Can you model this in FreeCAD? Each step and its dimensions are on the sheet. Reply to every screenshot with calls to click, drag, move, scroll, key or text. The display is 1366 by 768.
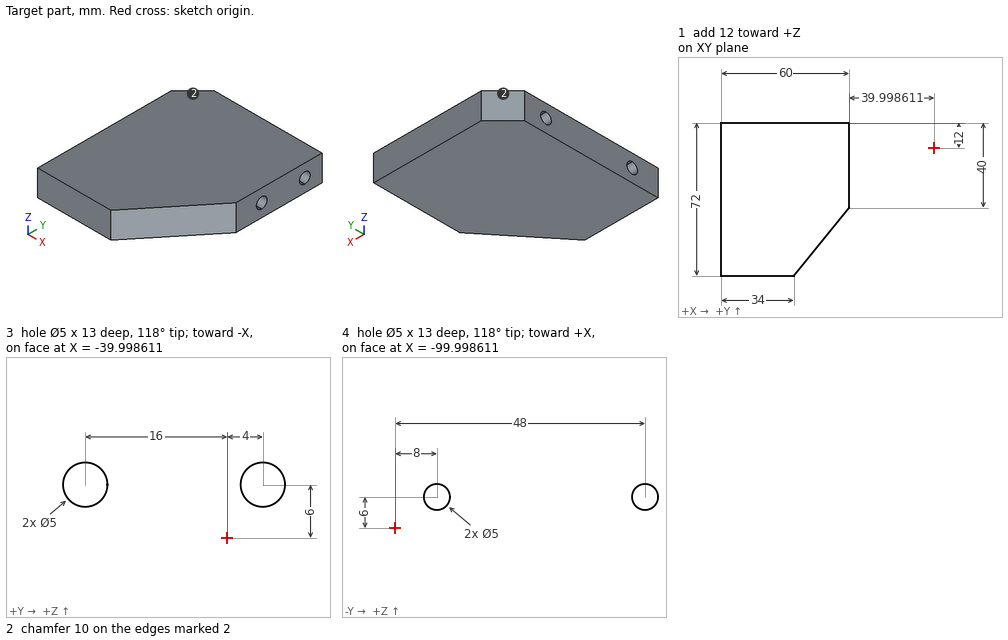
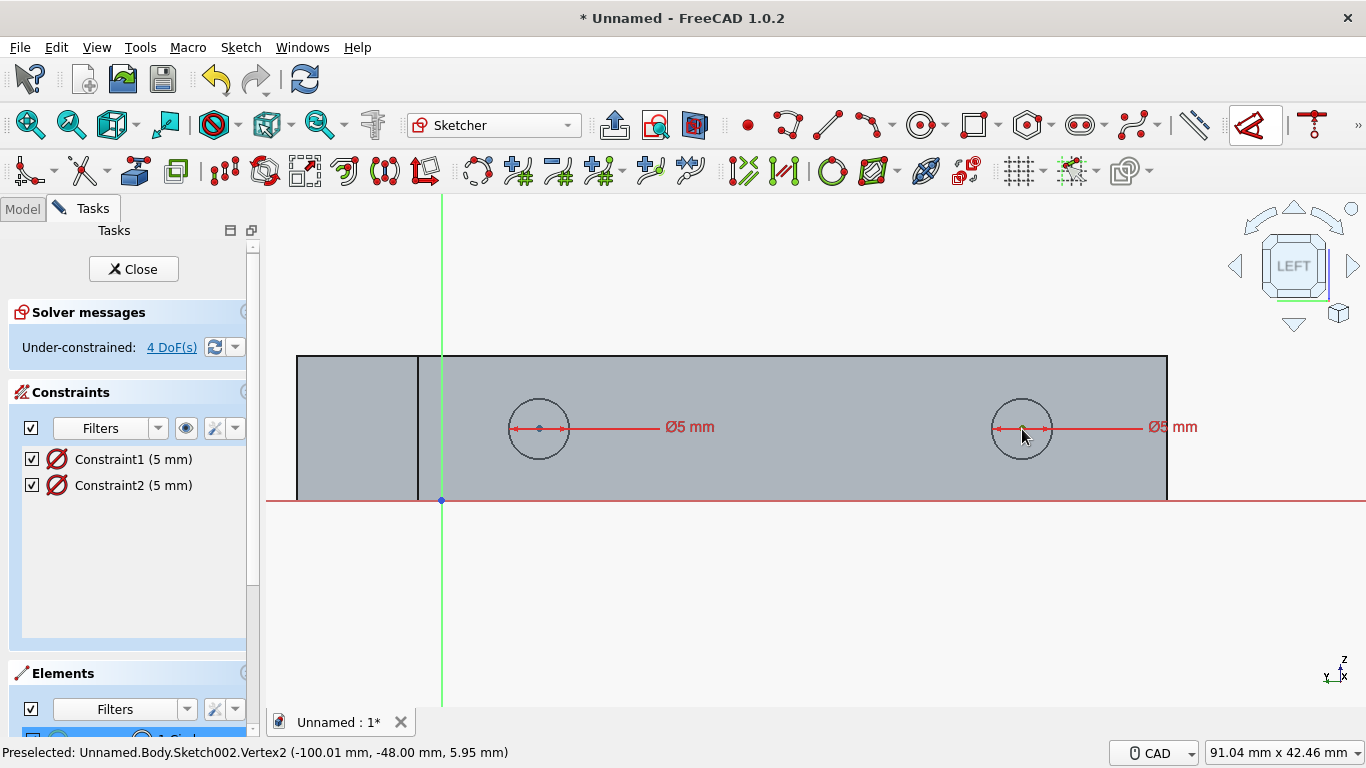
key(h)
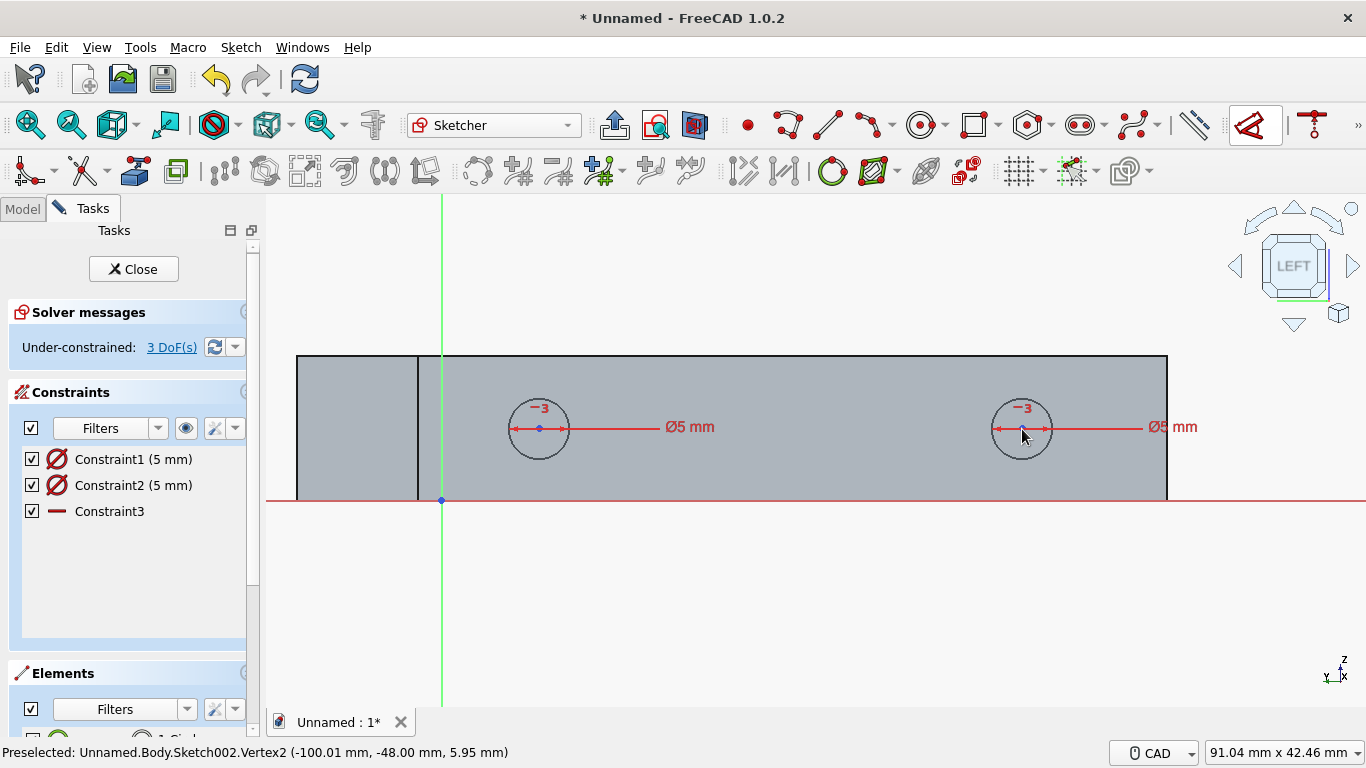
click(539, 429)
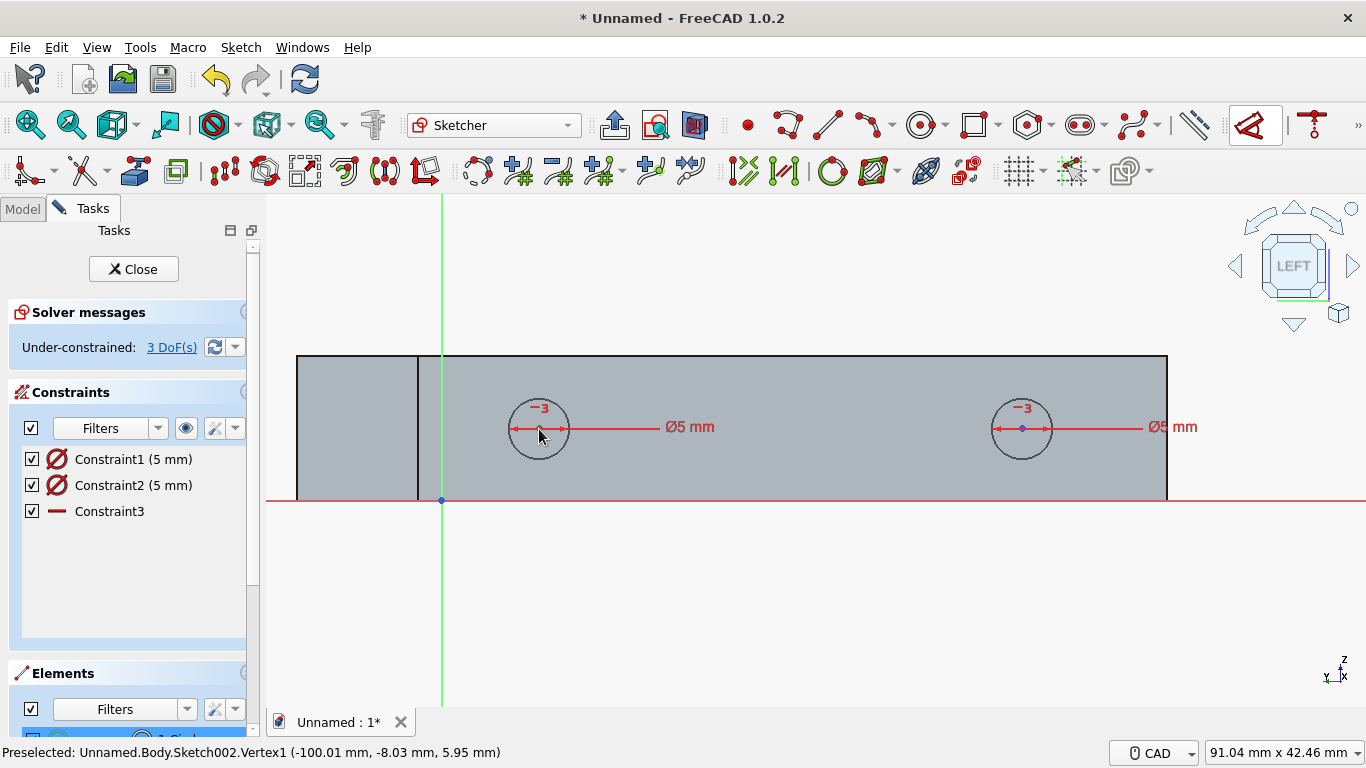
key(l)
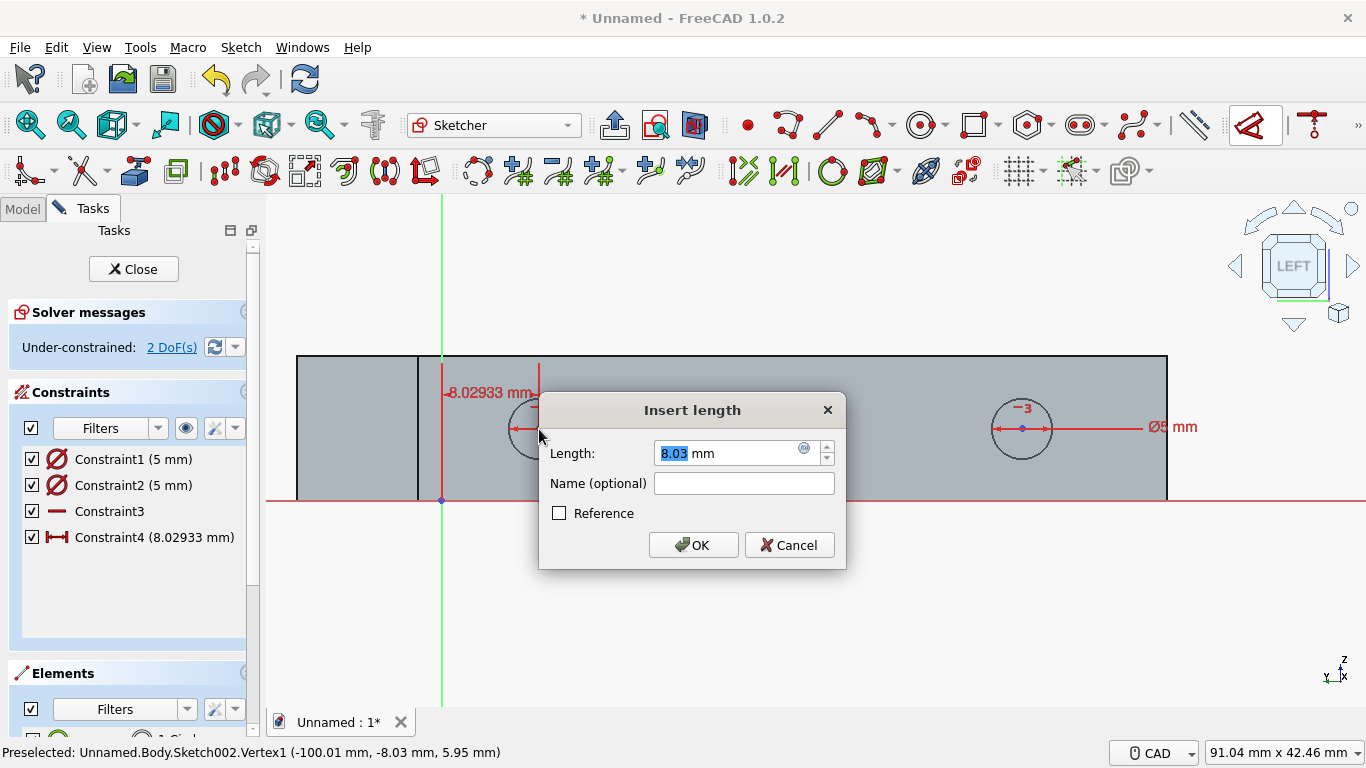
text(8)
key(Return)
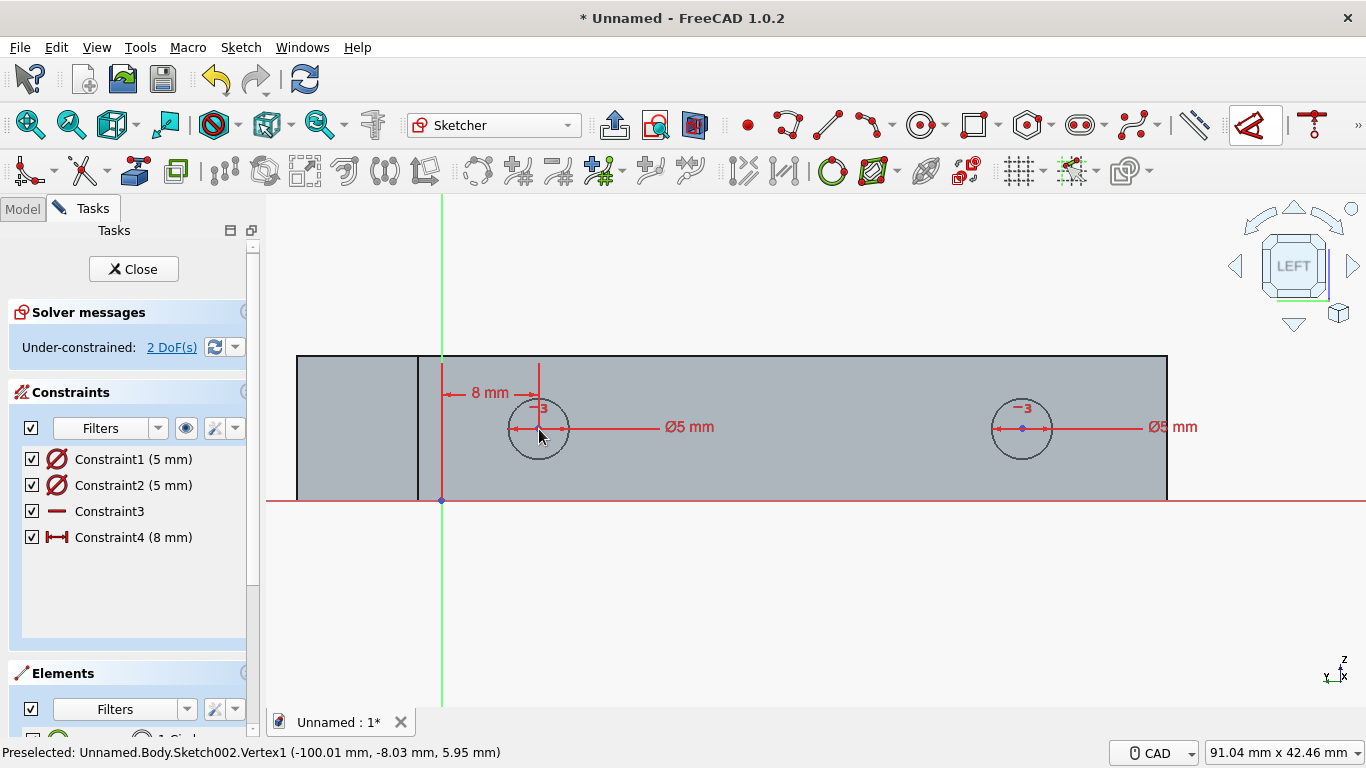
click(539, 429)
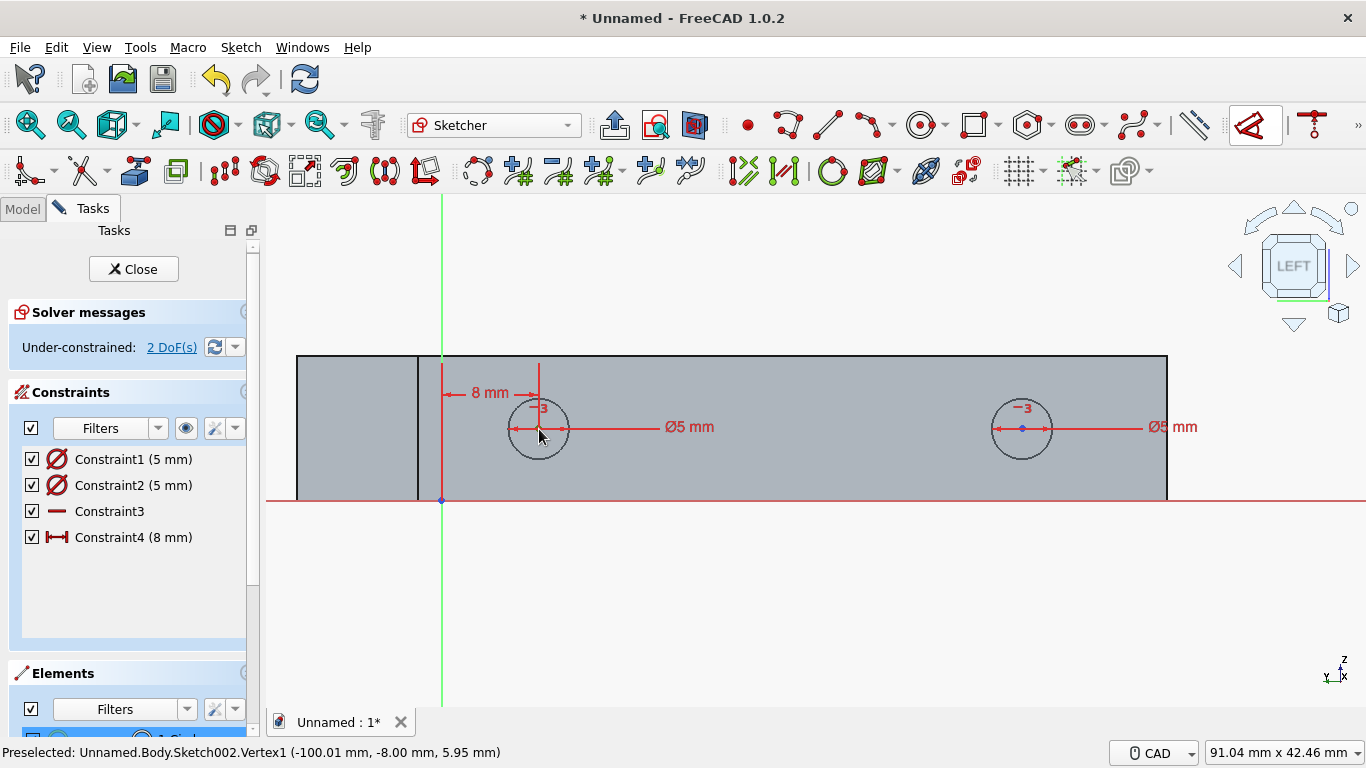
click(1276, 126)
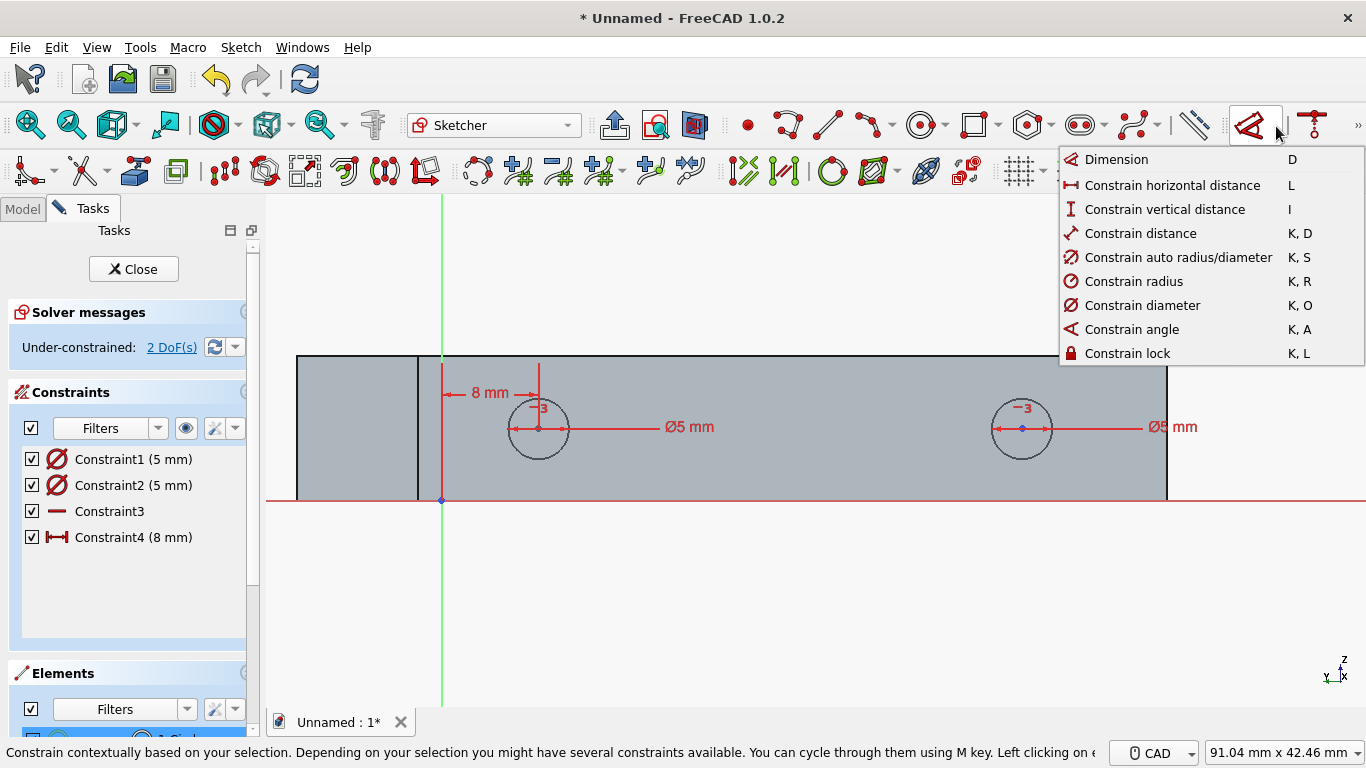
click(1212, 209)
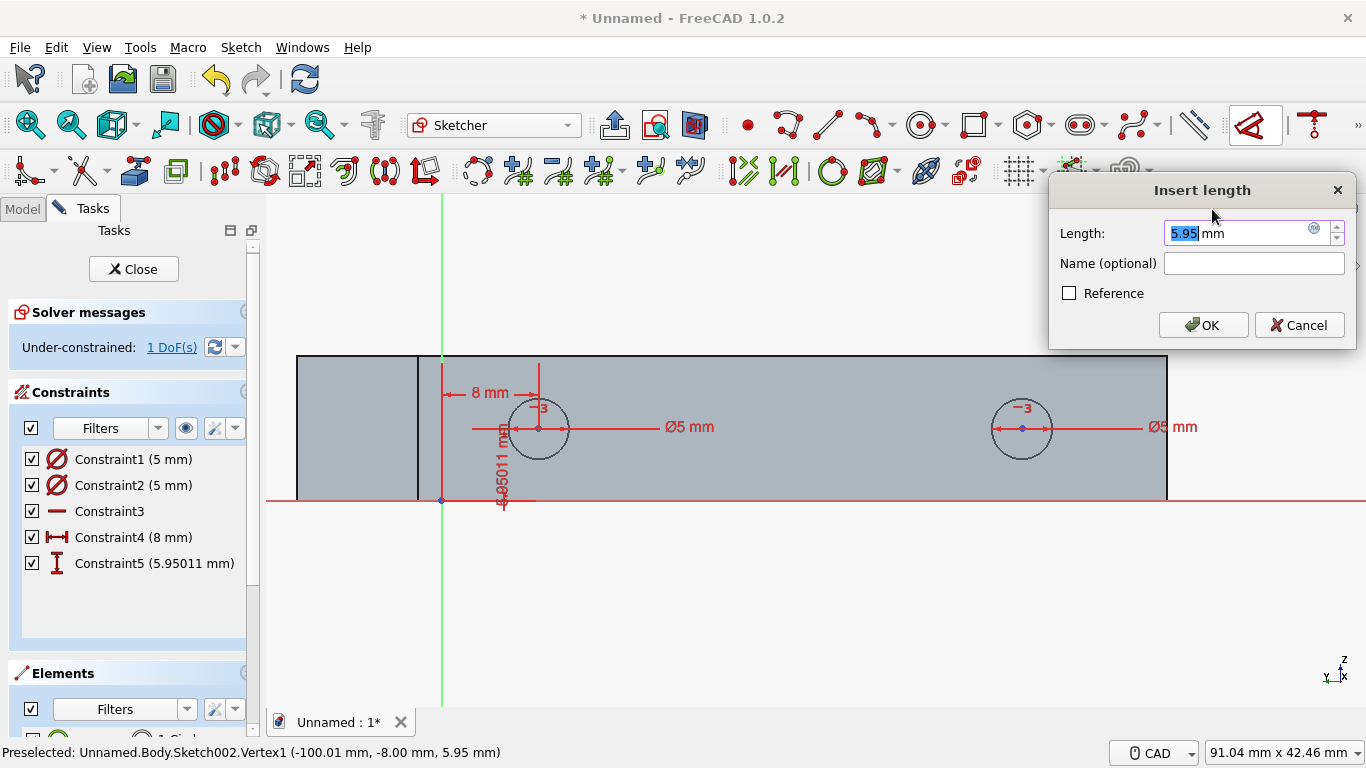
text(6)
key(Return)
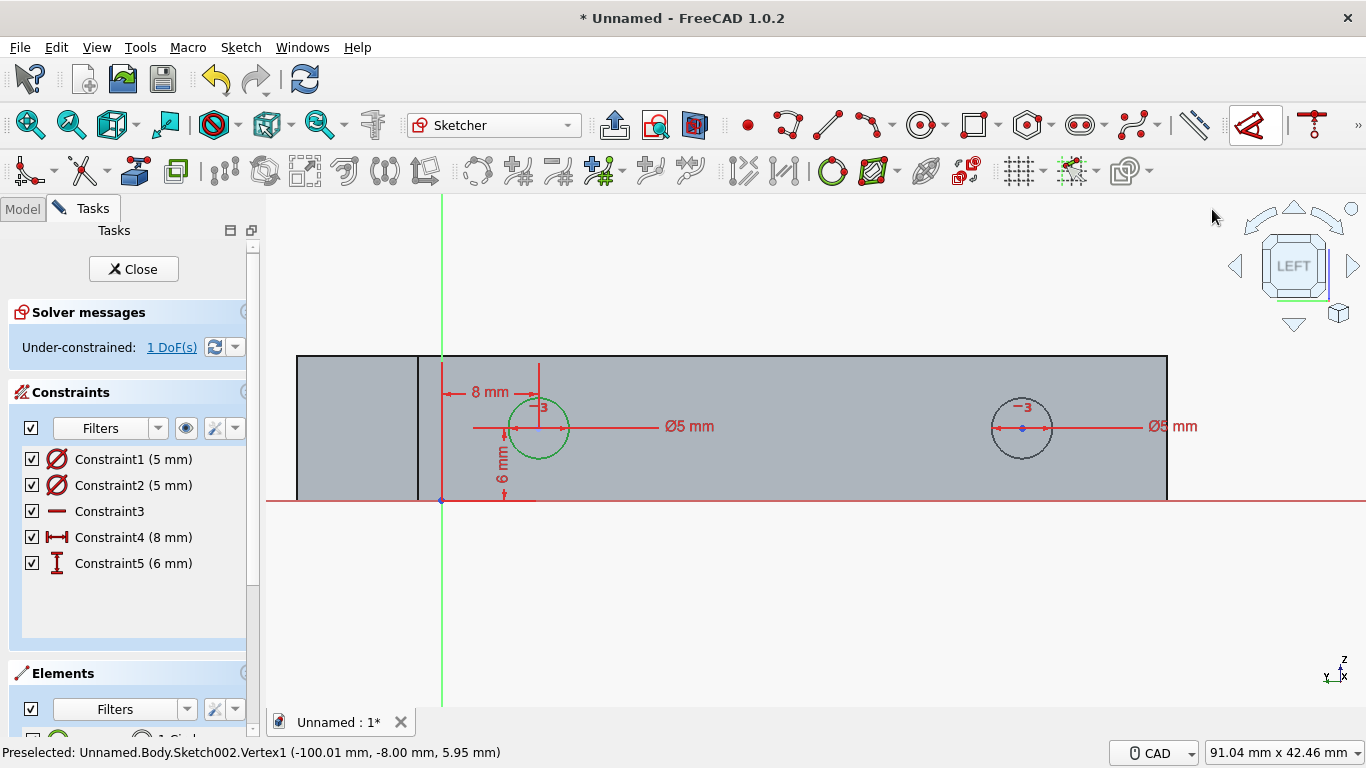
click(1022, 428)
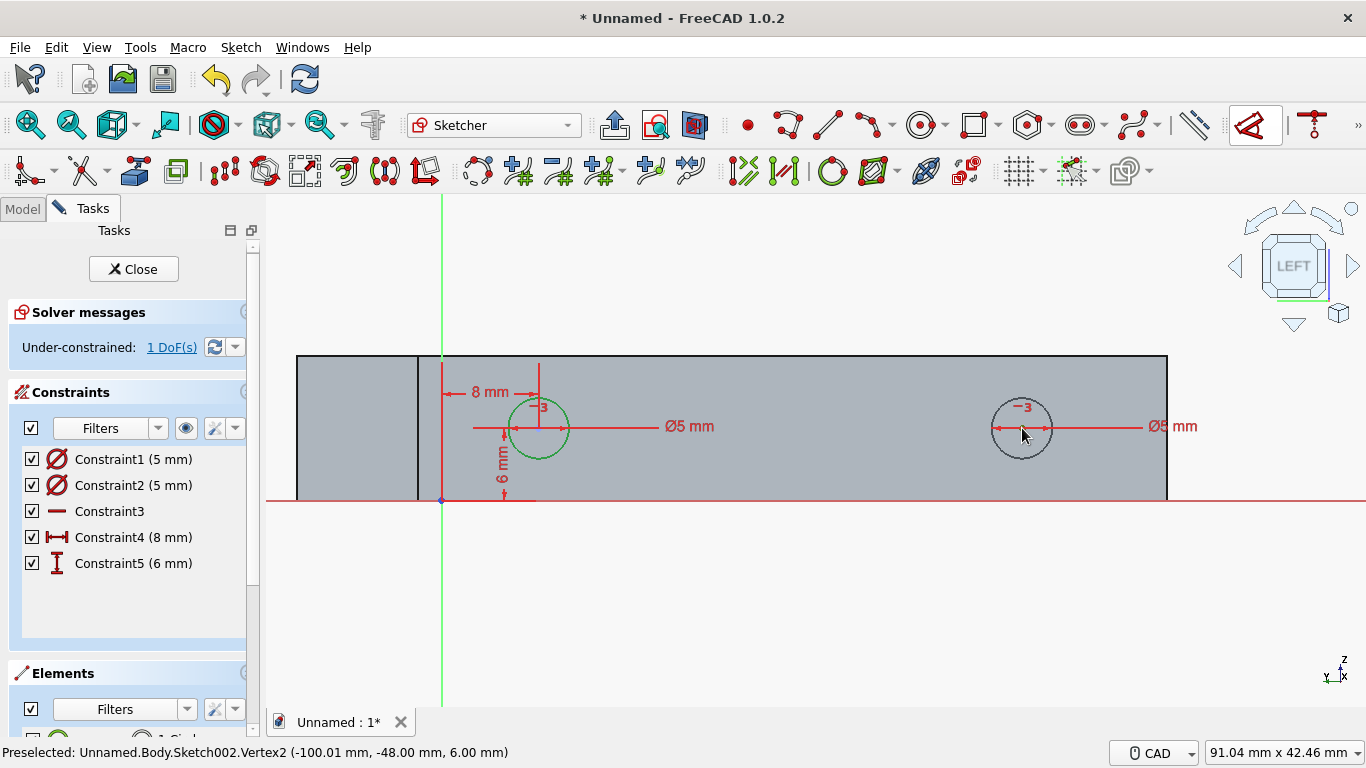
key(l)